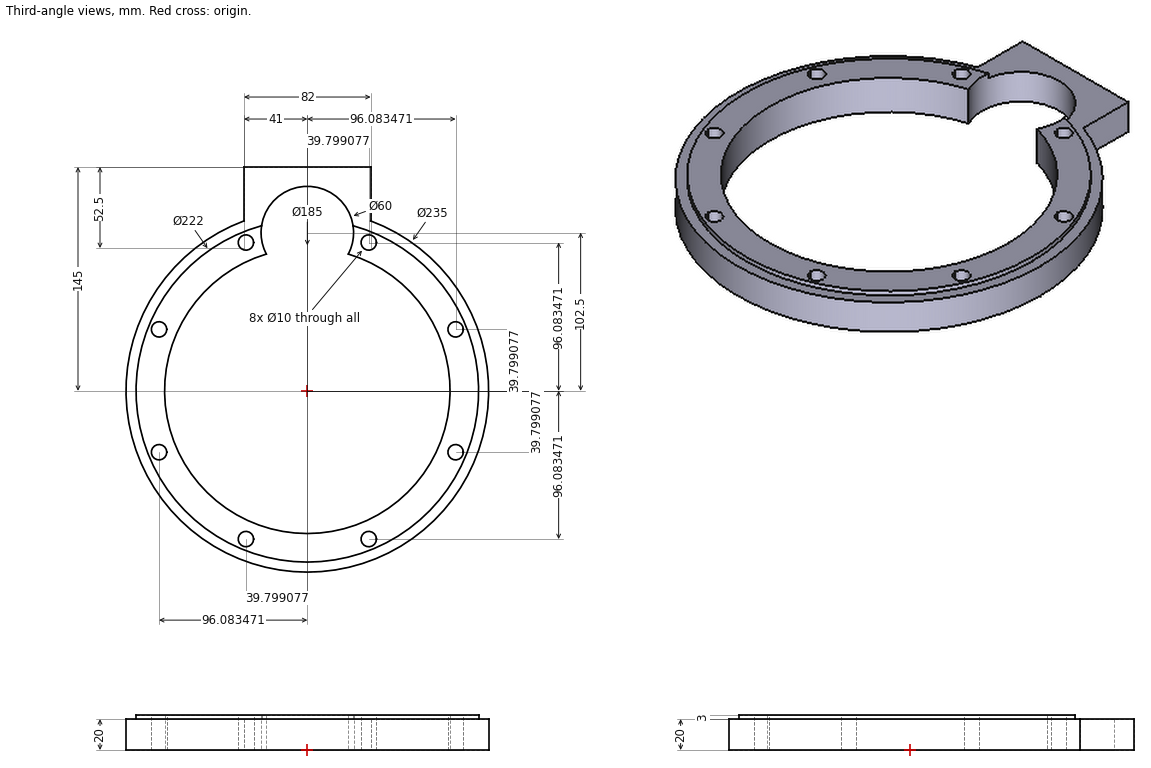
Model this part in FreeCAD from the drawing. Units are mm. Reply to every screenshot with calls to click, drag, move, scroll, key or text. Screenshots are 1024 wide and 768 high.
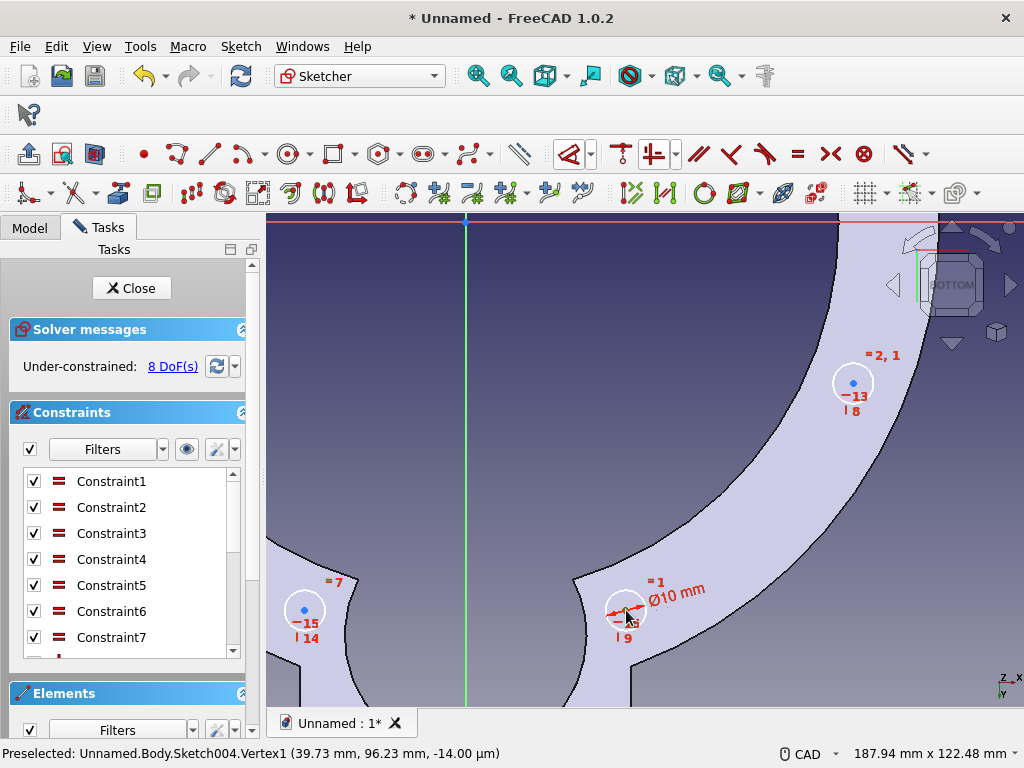
key(l)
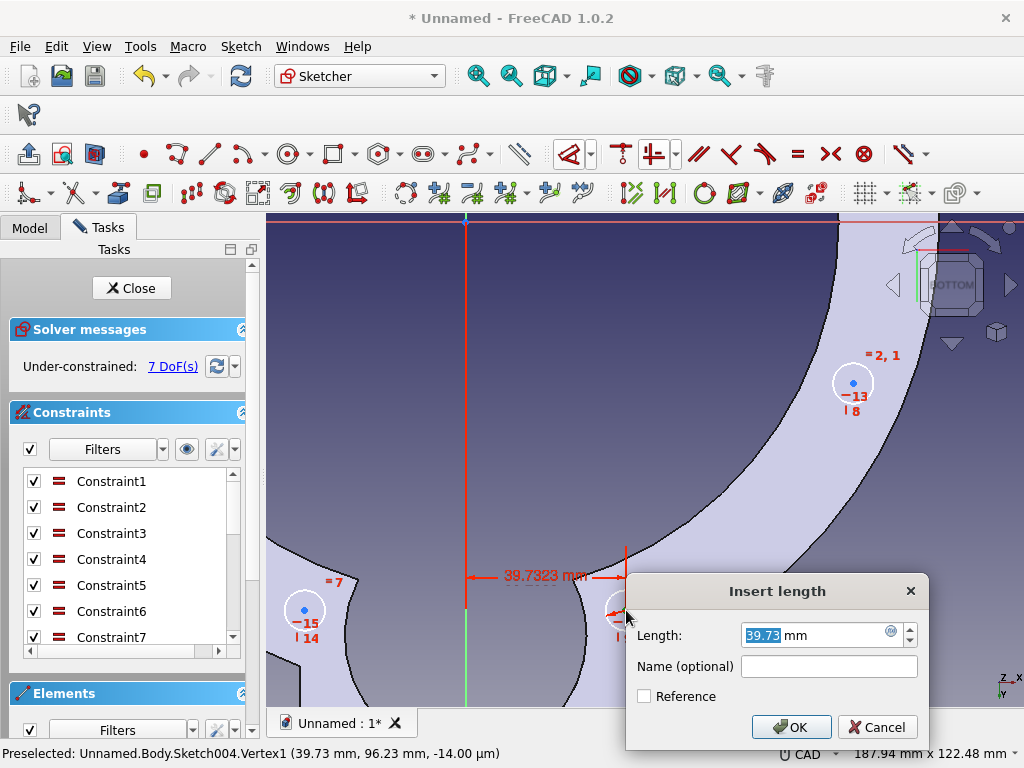
text(39.799077)
key(Return)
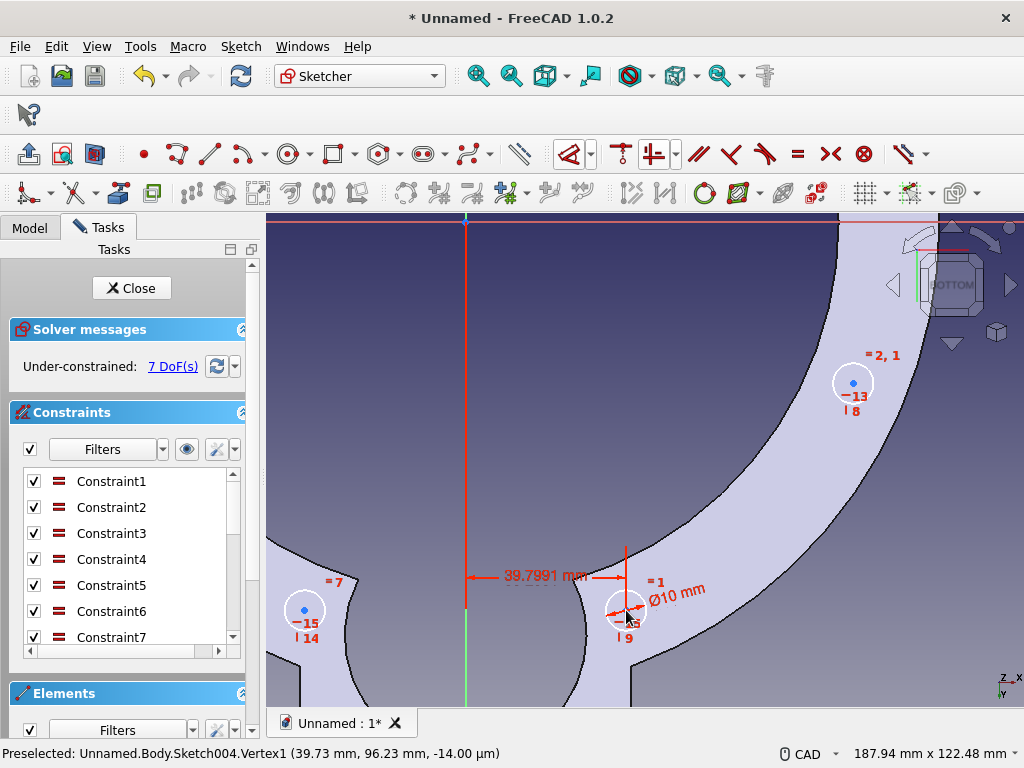
click(626, 610)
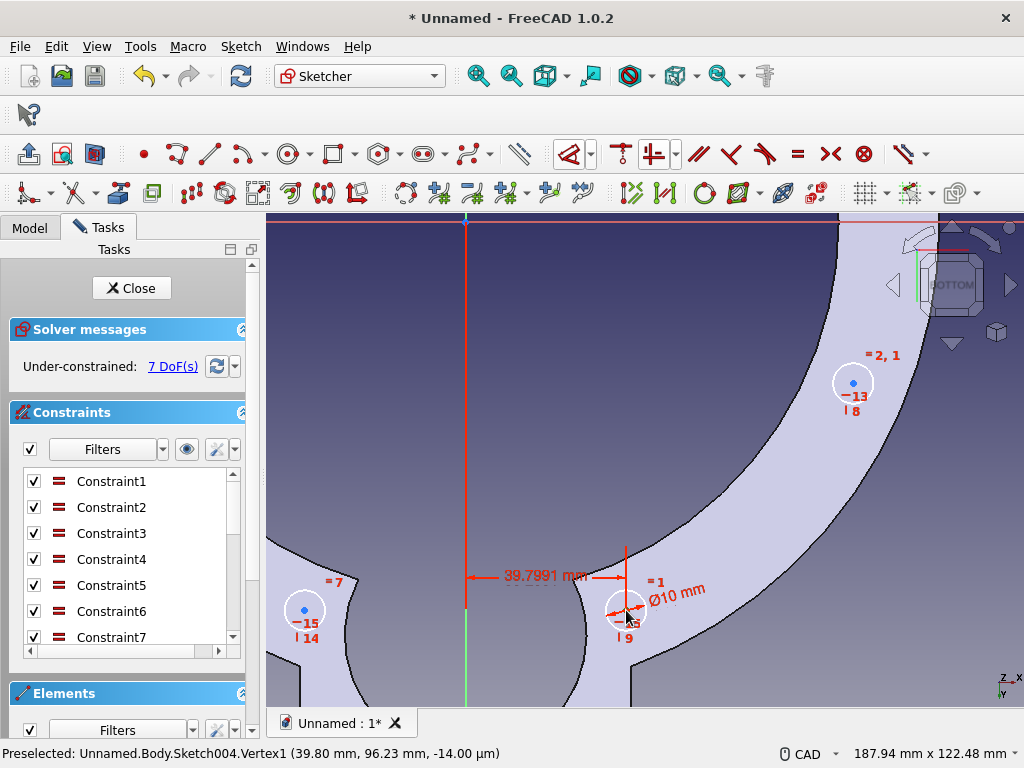
key(i)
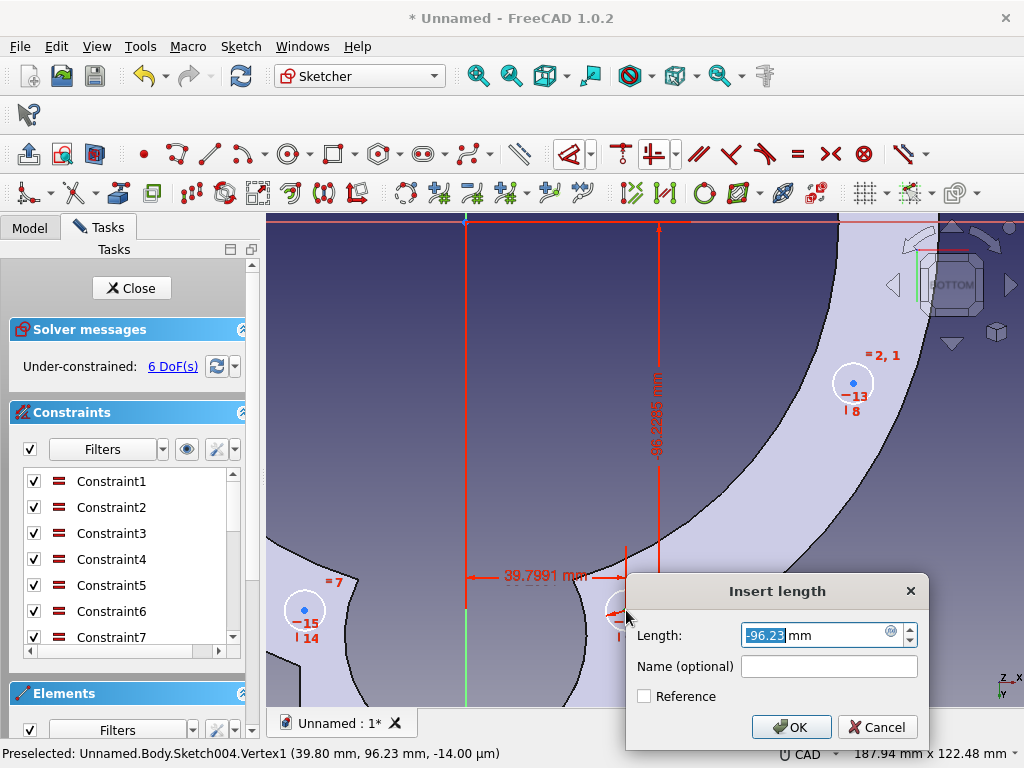
text(-96.083471)
key(Return)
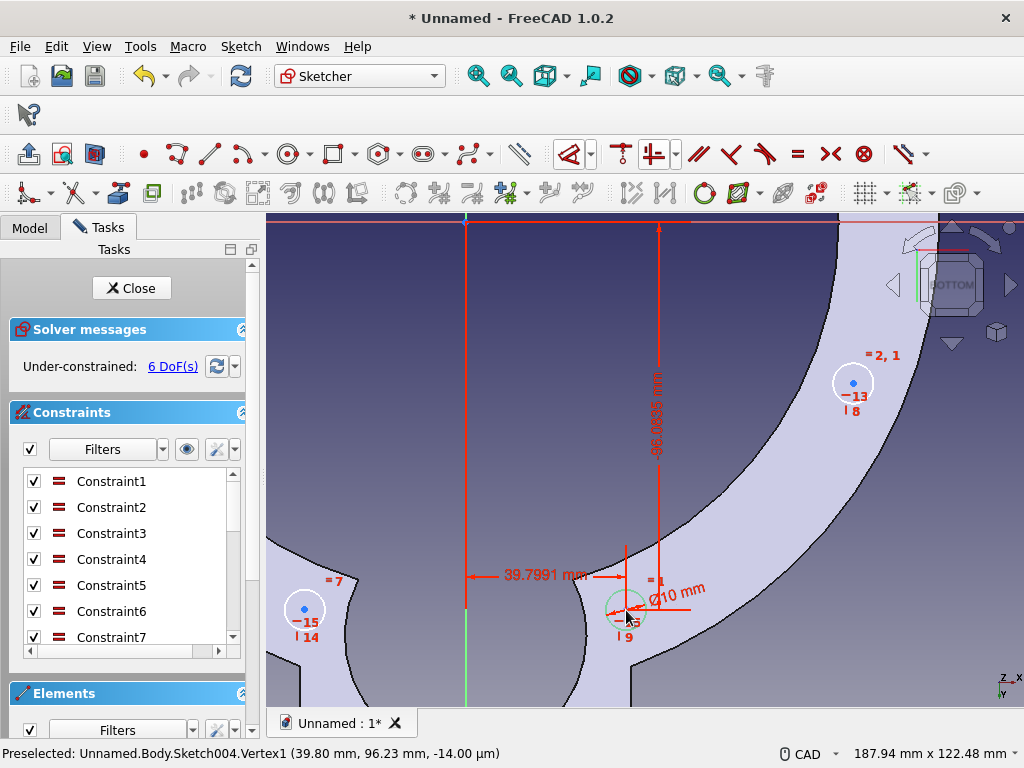
click(853, 383)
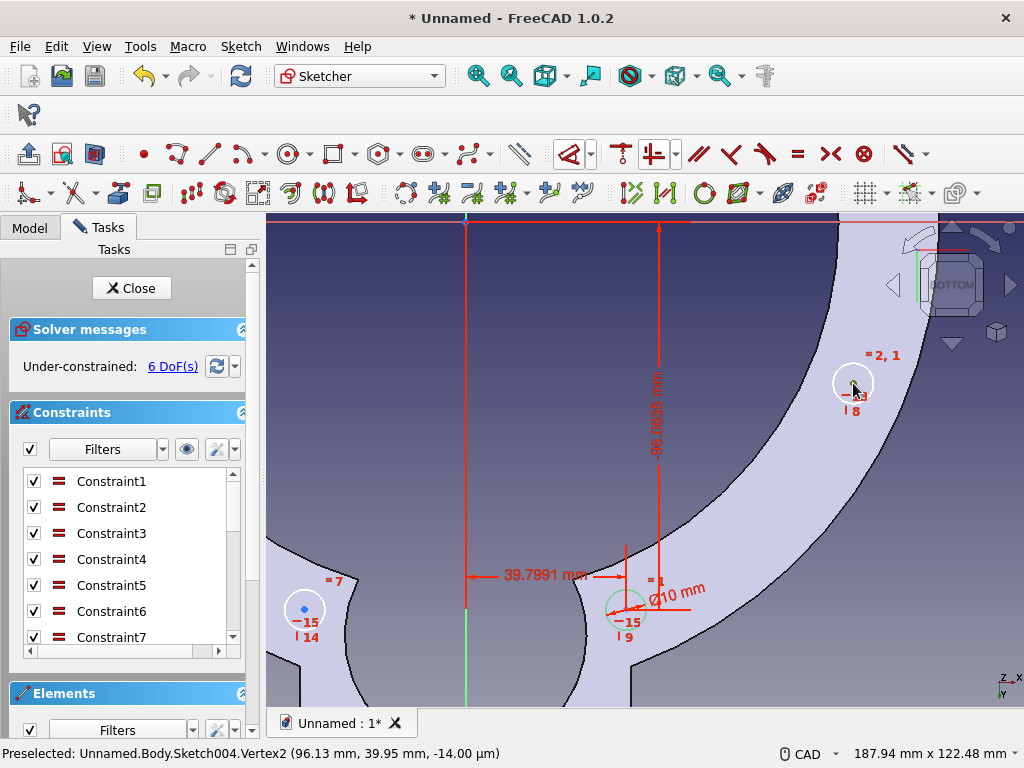
click(590, 154)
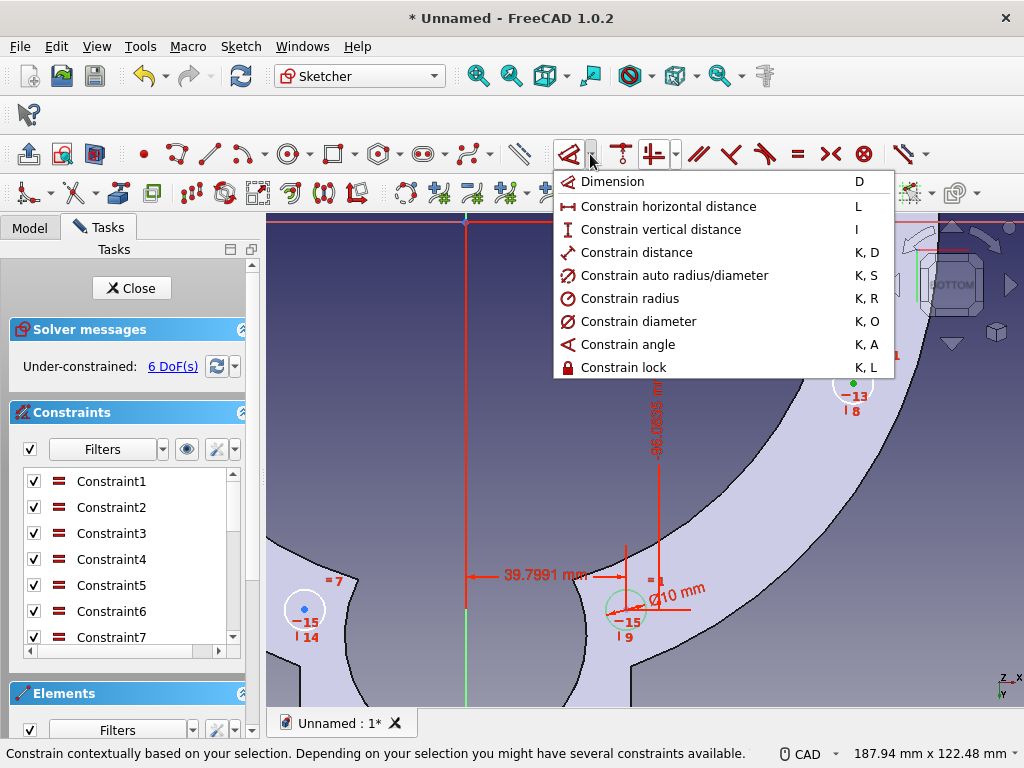
click(724, 206)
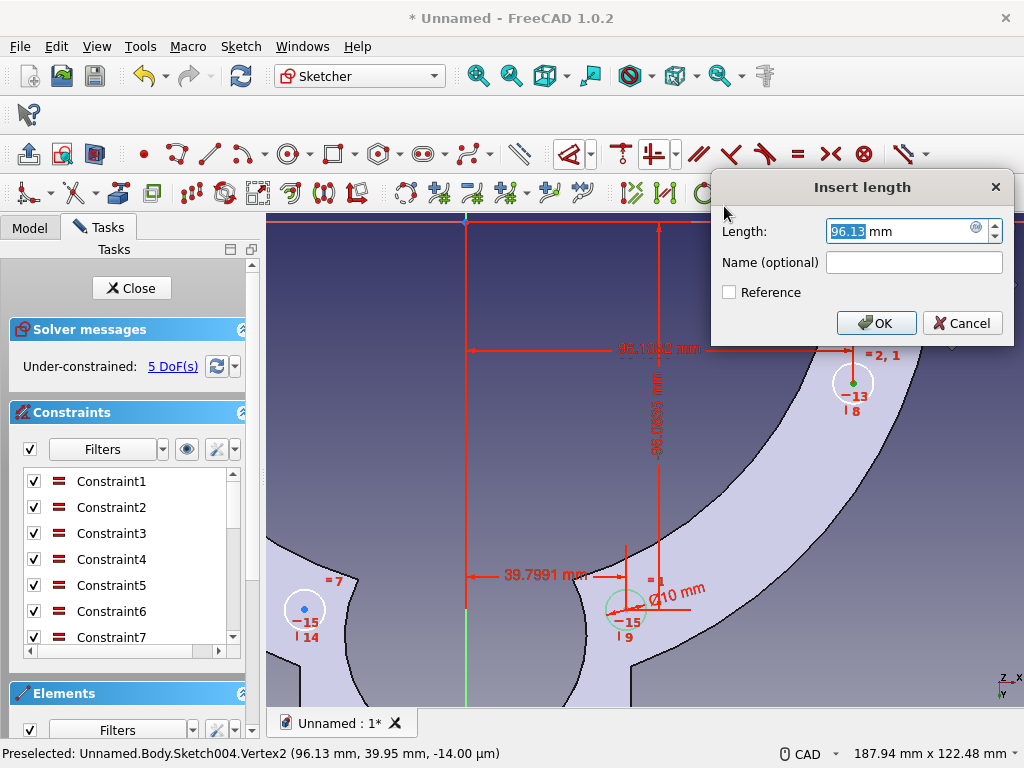
text(96.083471)
key(Return)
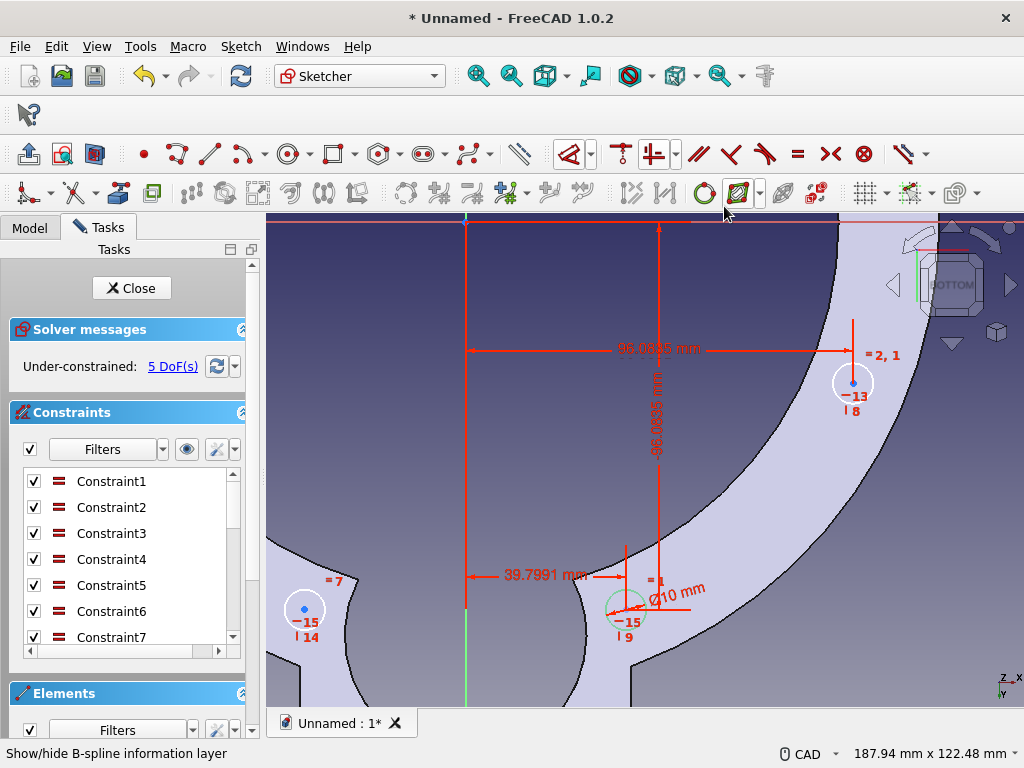
click(853, 383)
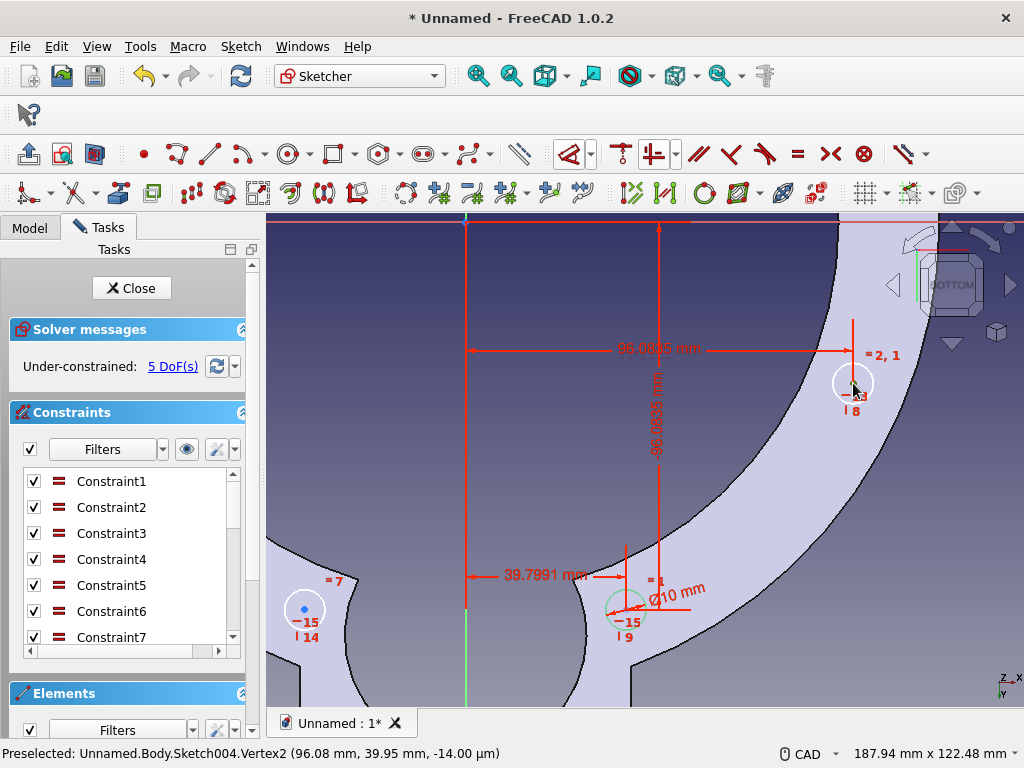
key(i)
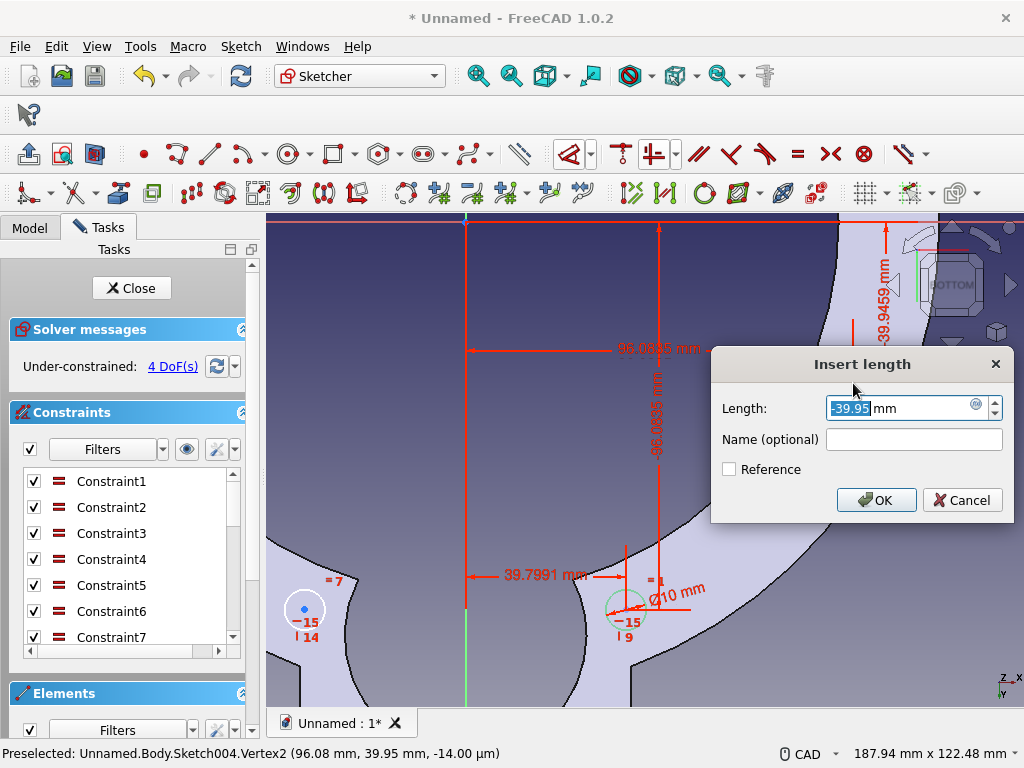
text(-39.799077)
key(Return)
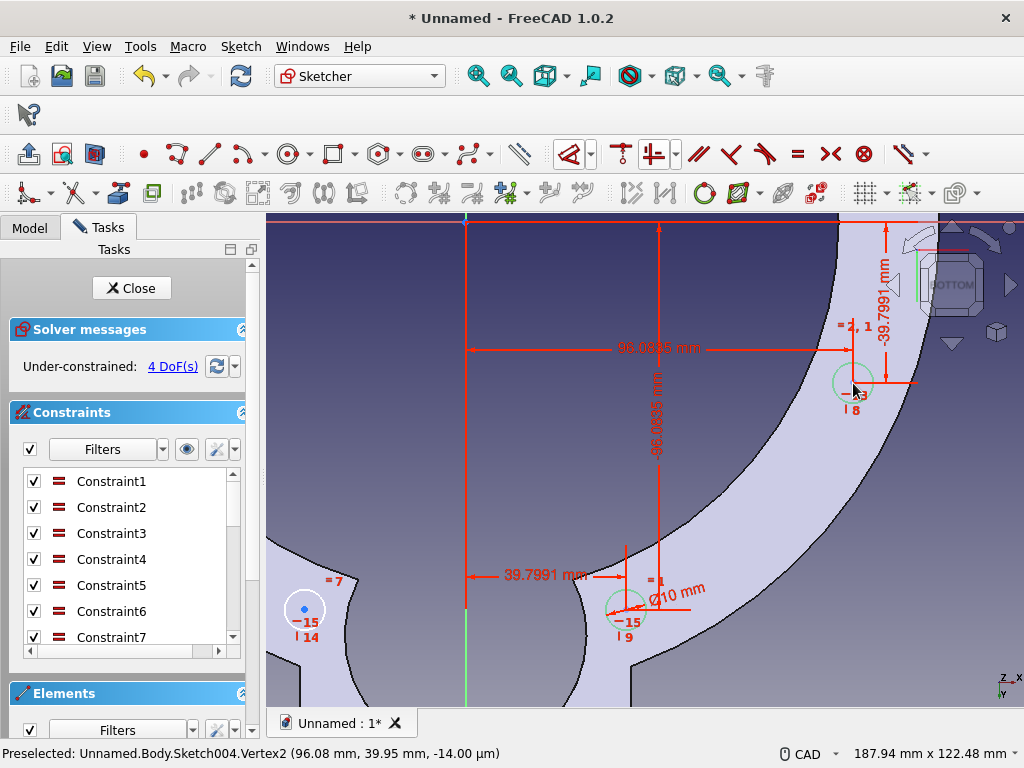
scroll(641, 598, down, 5)